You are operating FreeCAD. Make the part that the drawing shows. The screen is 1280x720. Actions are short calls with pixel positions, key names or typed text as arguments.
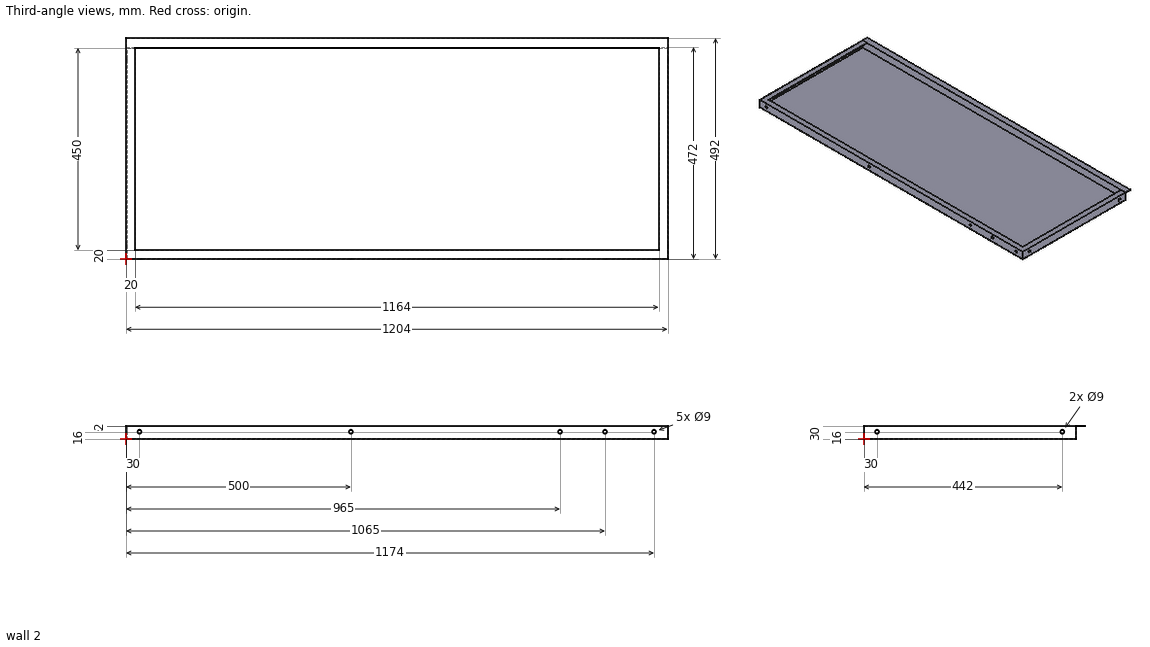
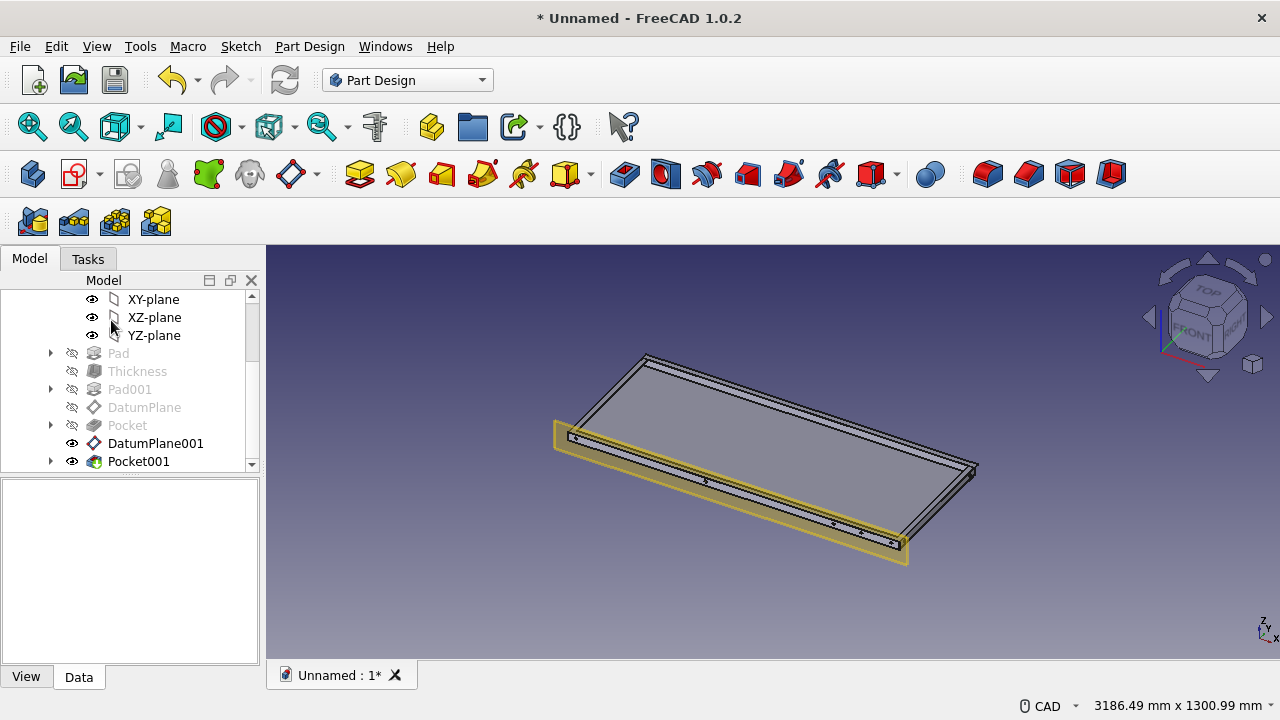
click(117, 443)
key(space)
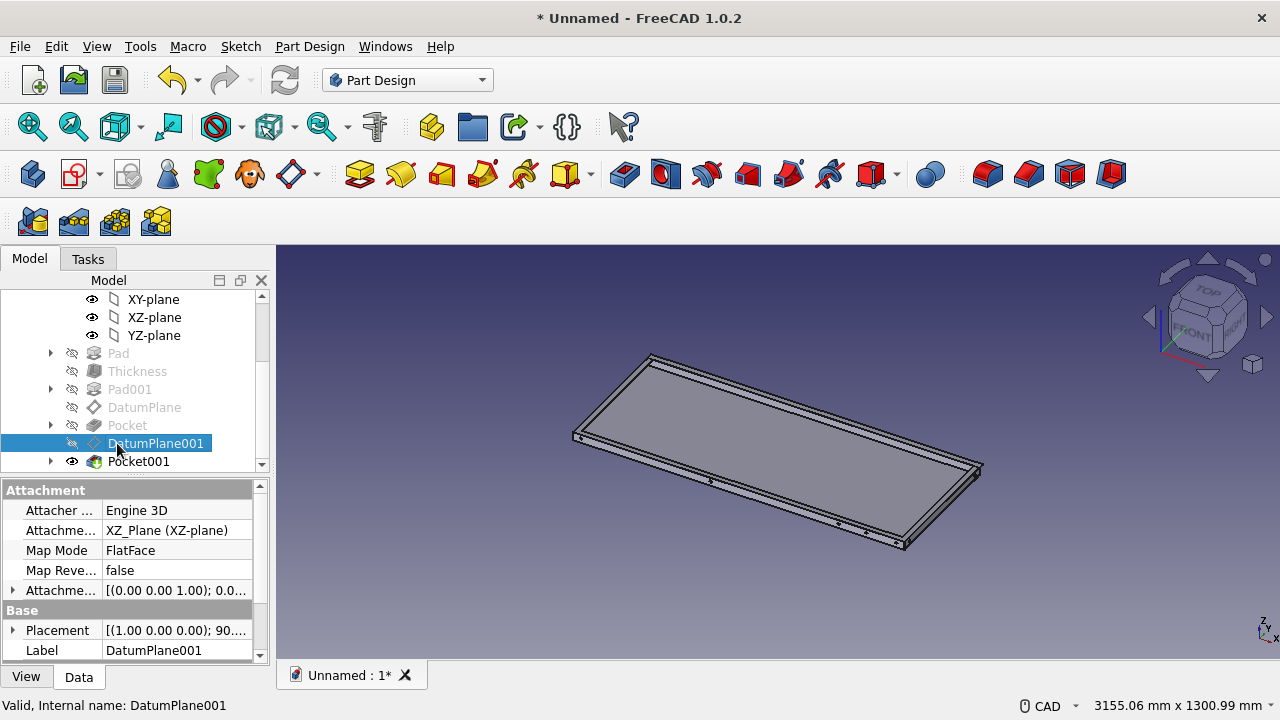
key(0)